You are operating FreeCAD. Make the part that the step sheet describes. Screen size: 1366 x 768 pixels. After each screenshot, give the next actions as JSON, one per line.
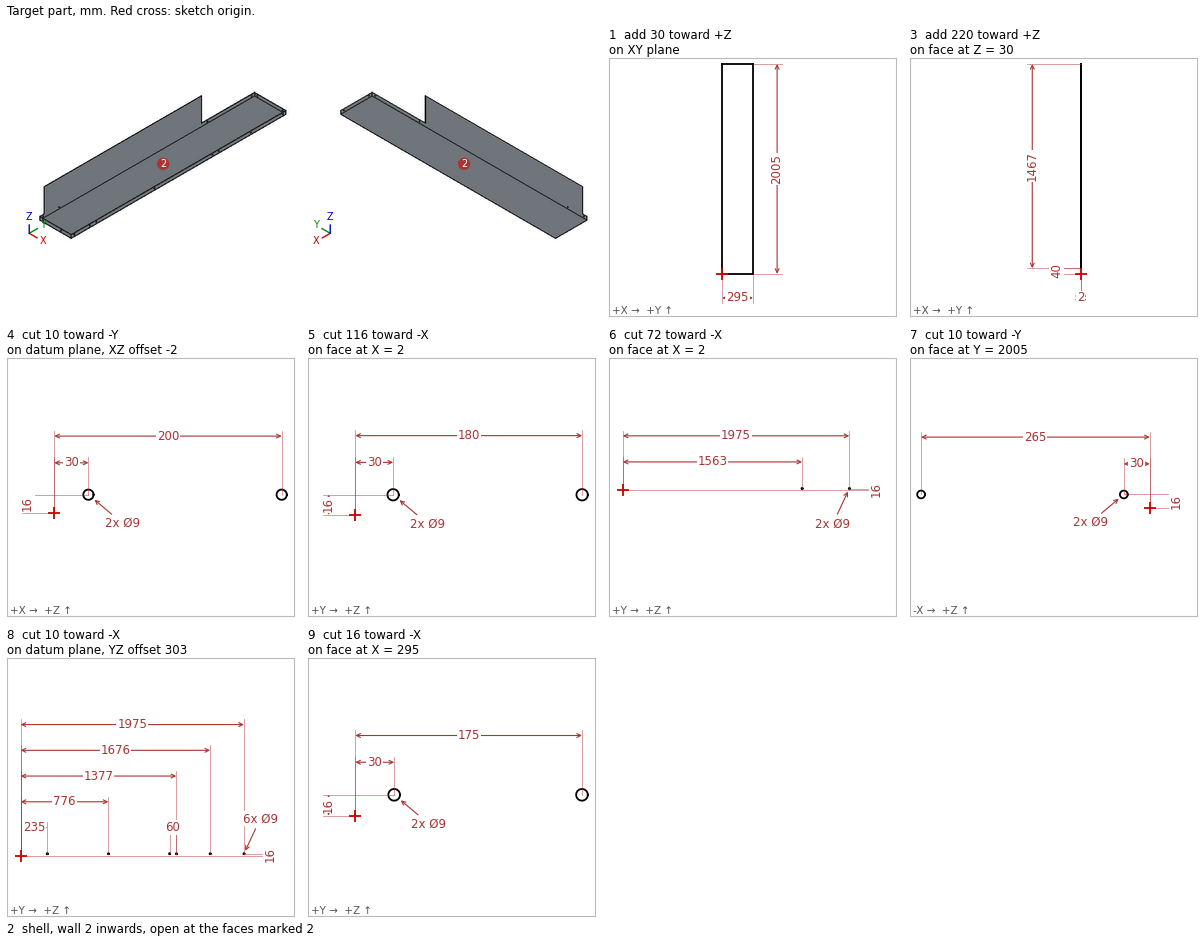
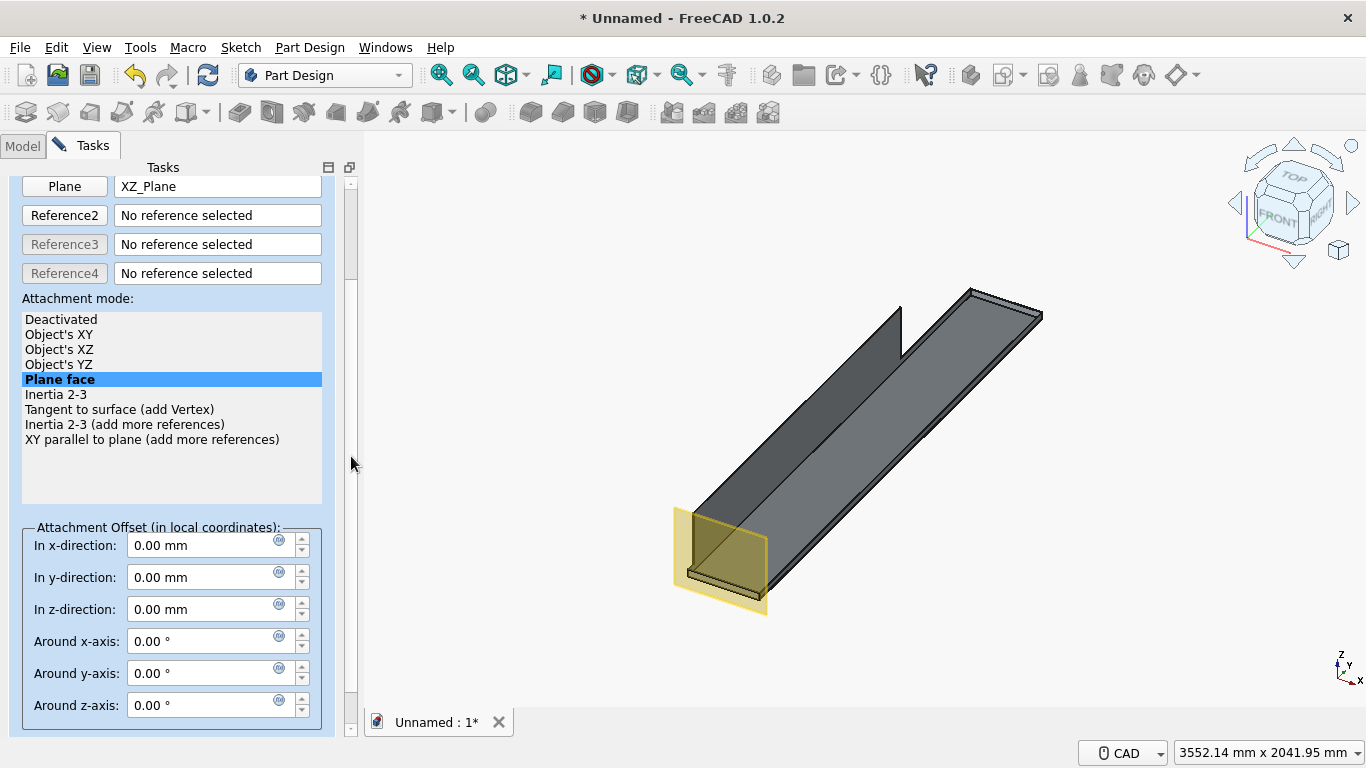
{"action": "triple_click", "coordinate": [210, 609]}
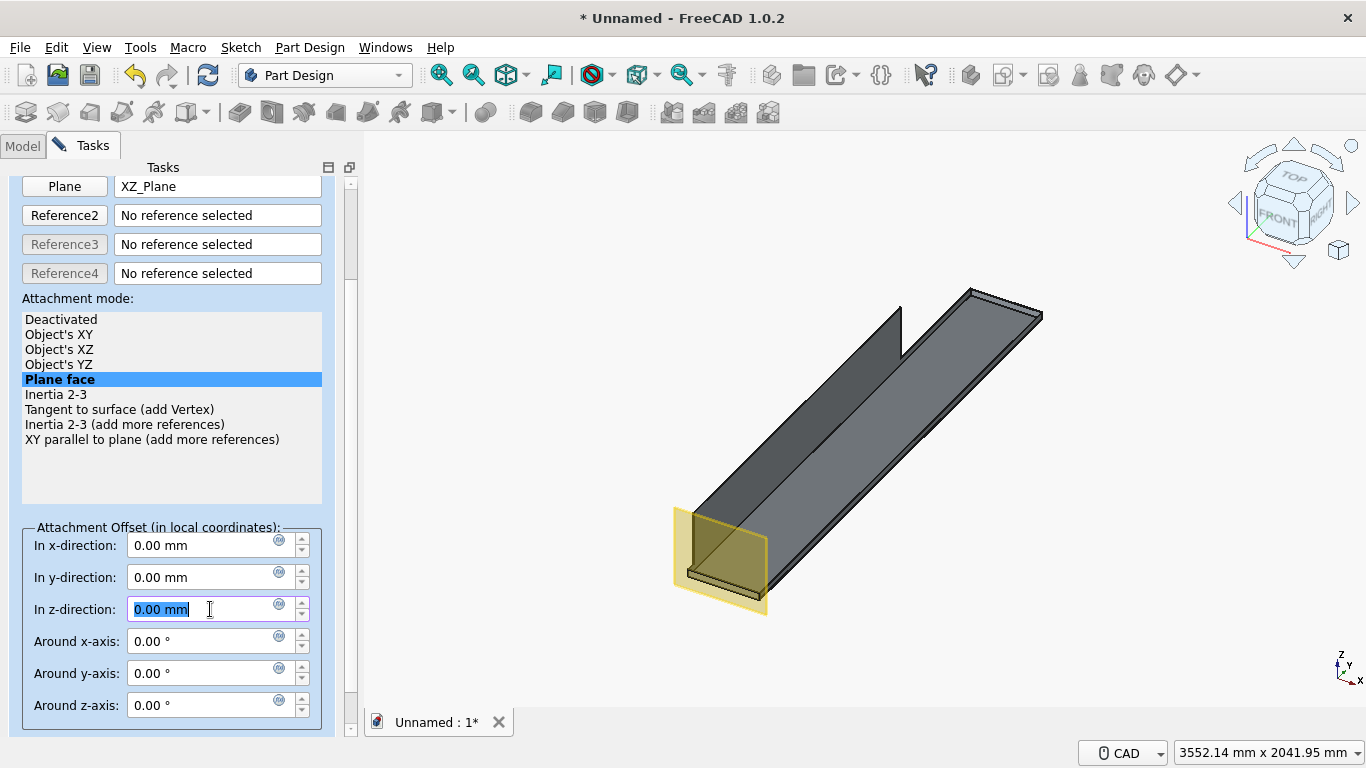
{"action": "type", "text": "-2"}
{"action": "key", "text": "Tab"}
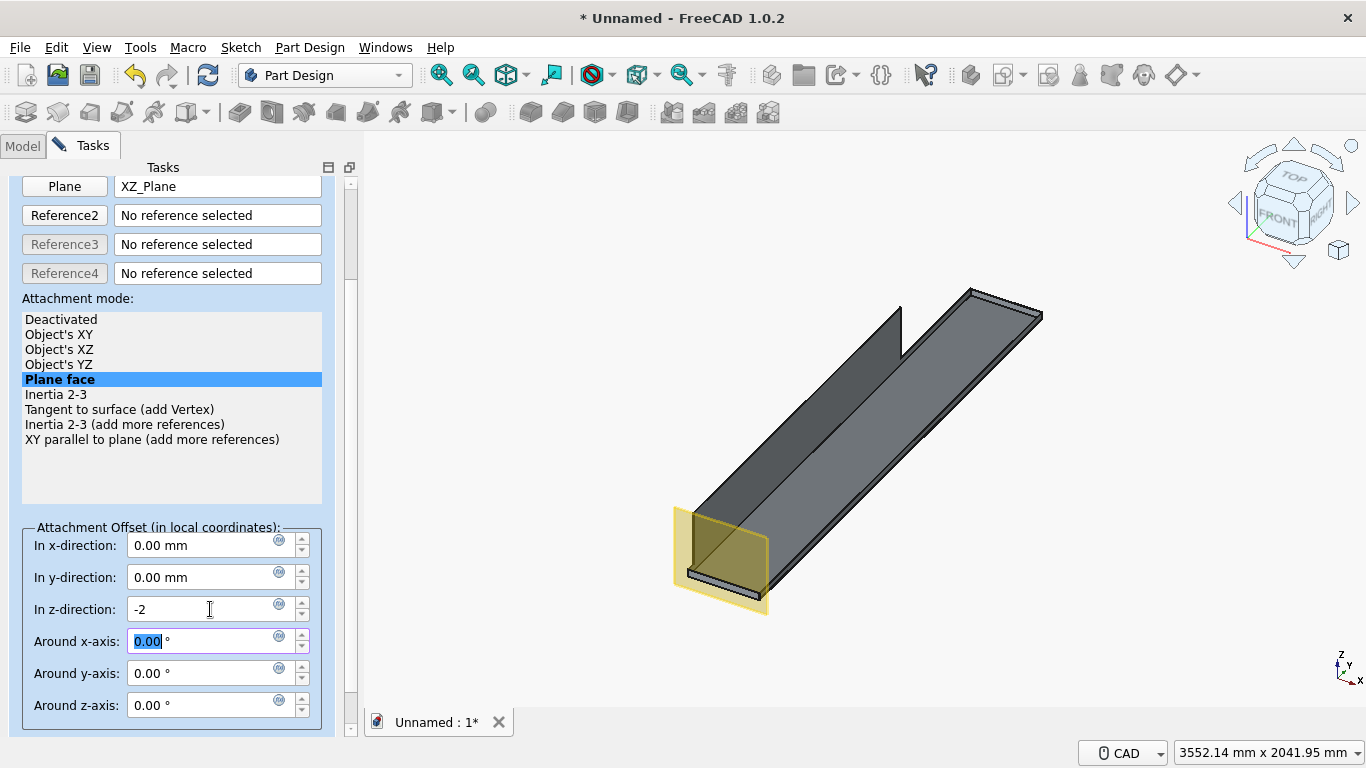
{"action": "scroll", "coordinate": [351, 456], "scroll_direction": "up", "scroll_amount": 3}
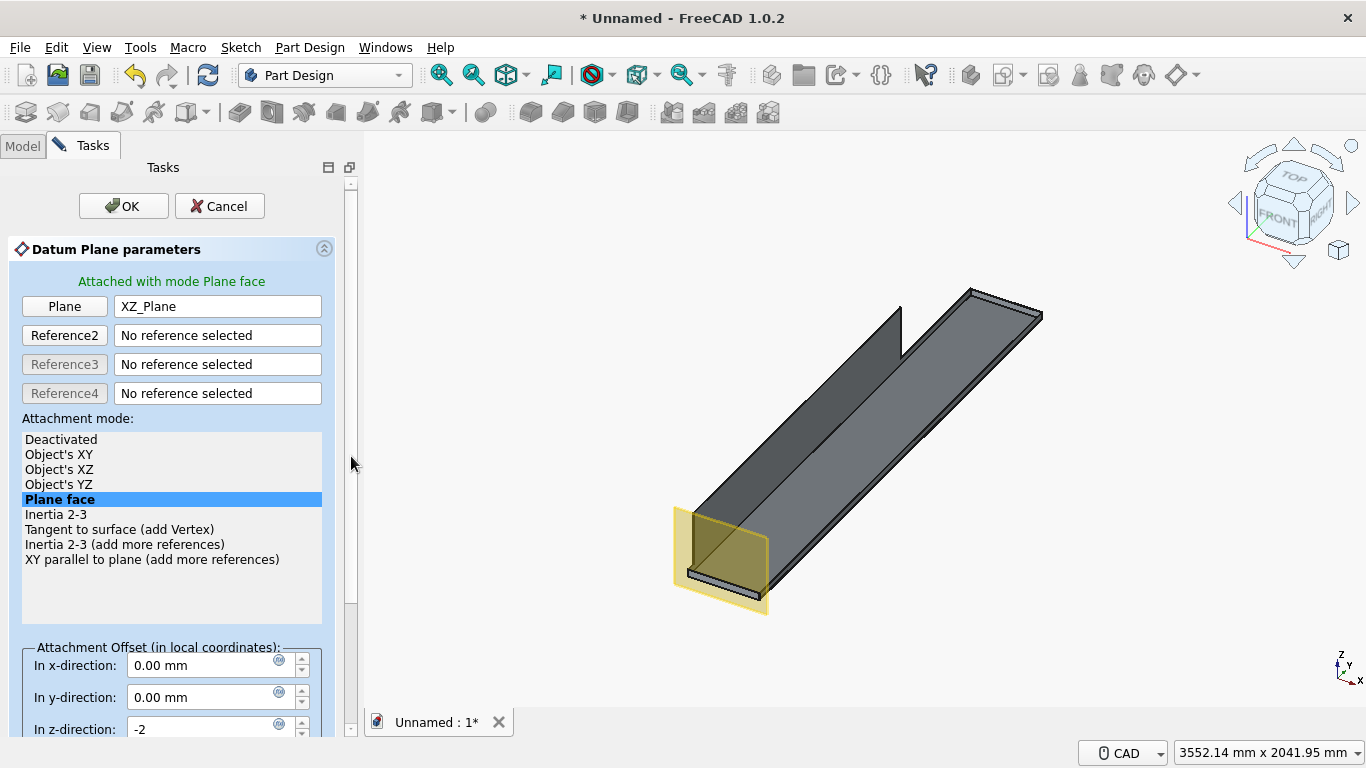
{"action": "left_click", "coordinate": [124, 206]}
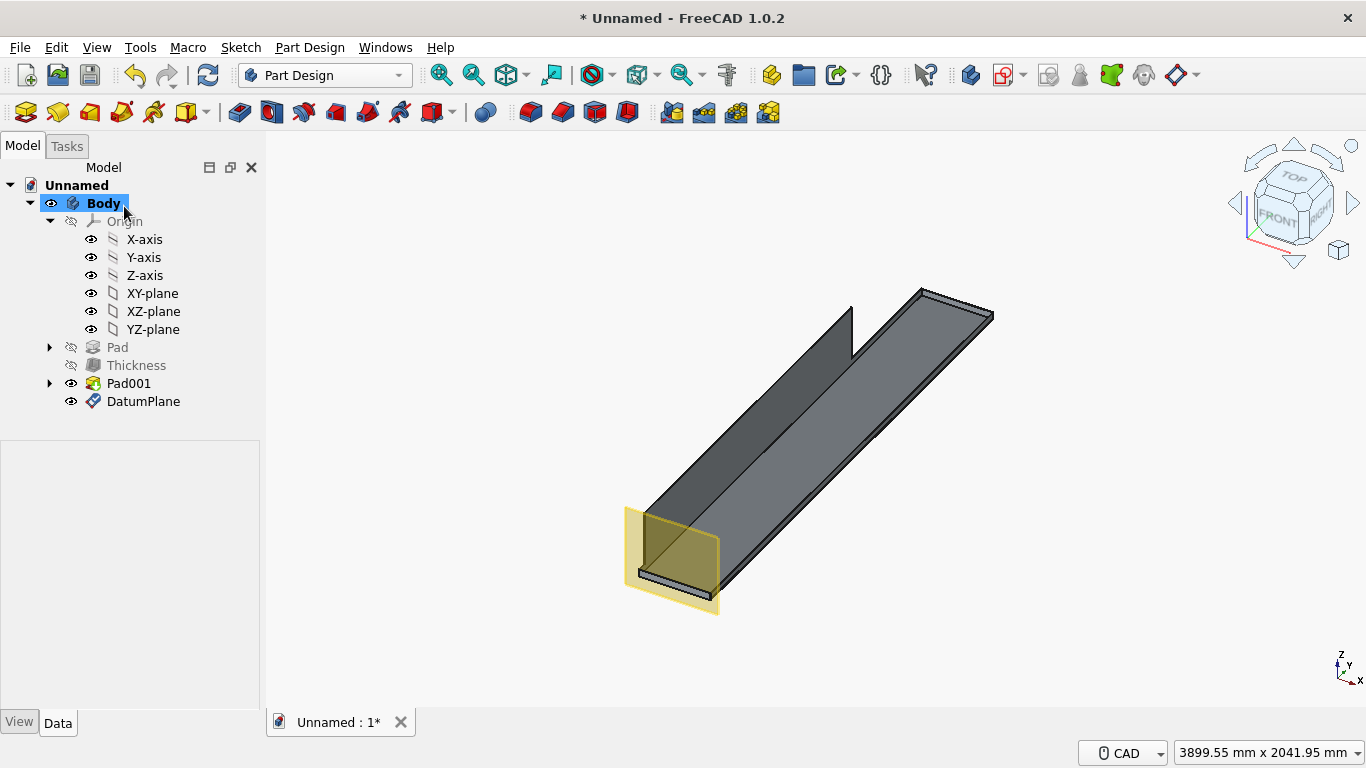
{"action": "left_click", "coordinate": [116, 401]}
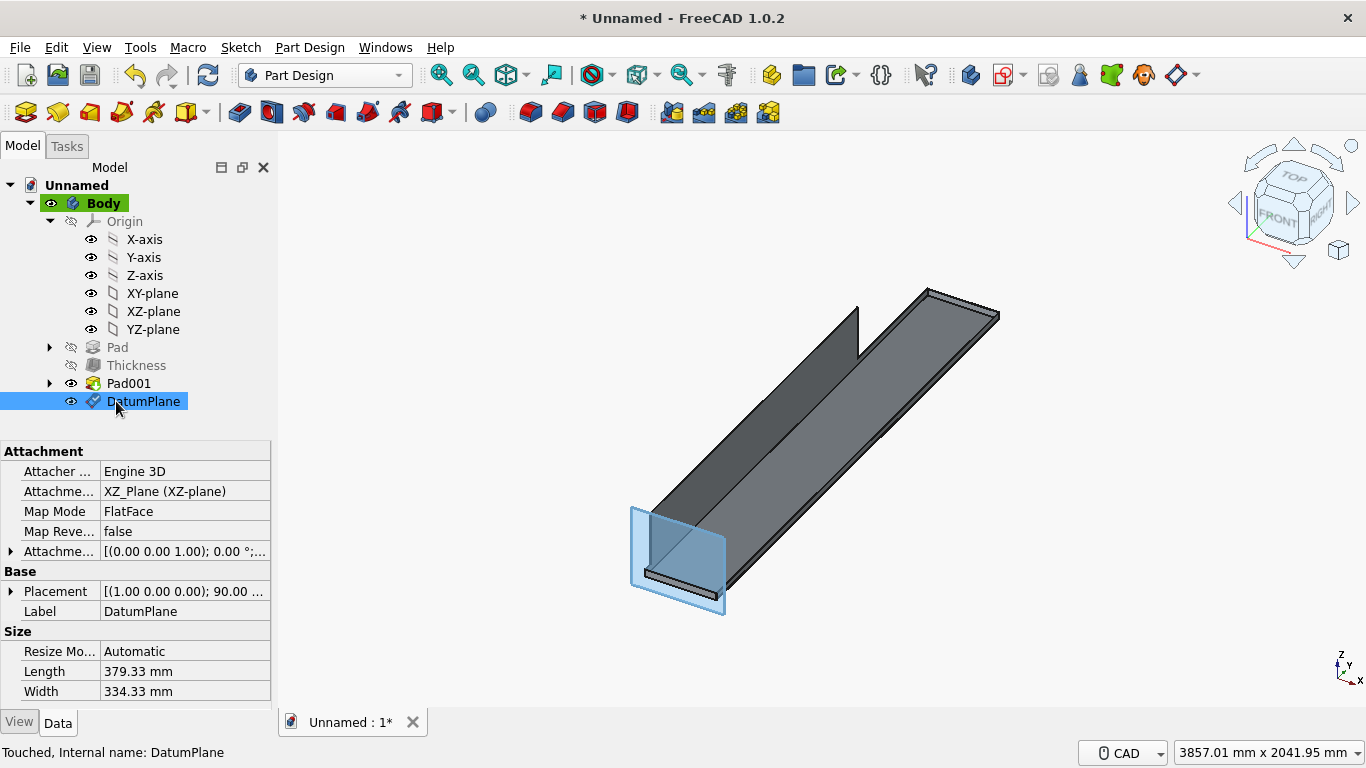
{"action": "left_click", "coordinate": [1004, 76]}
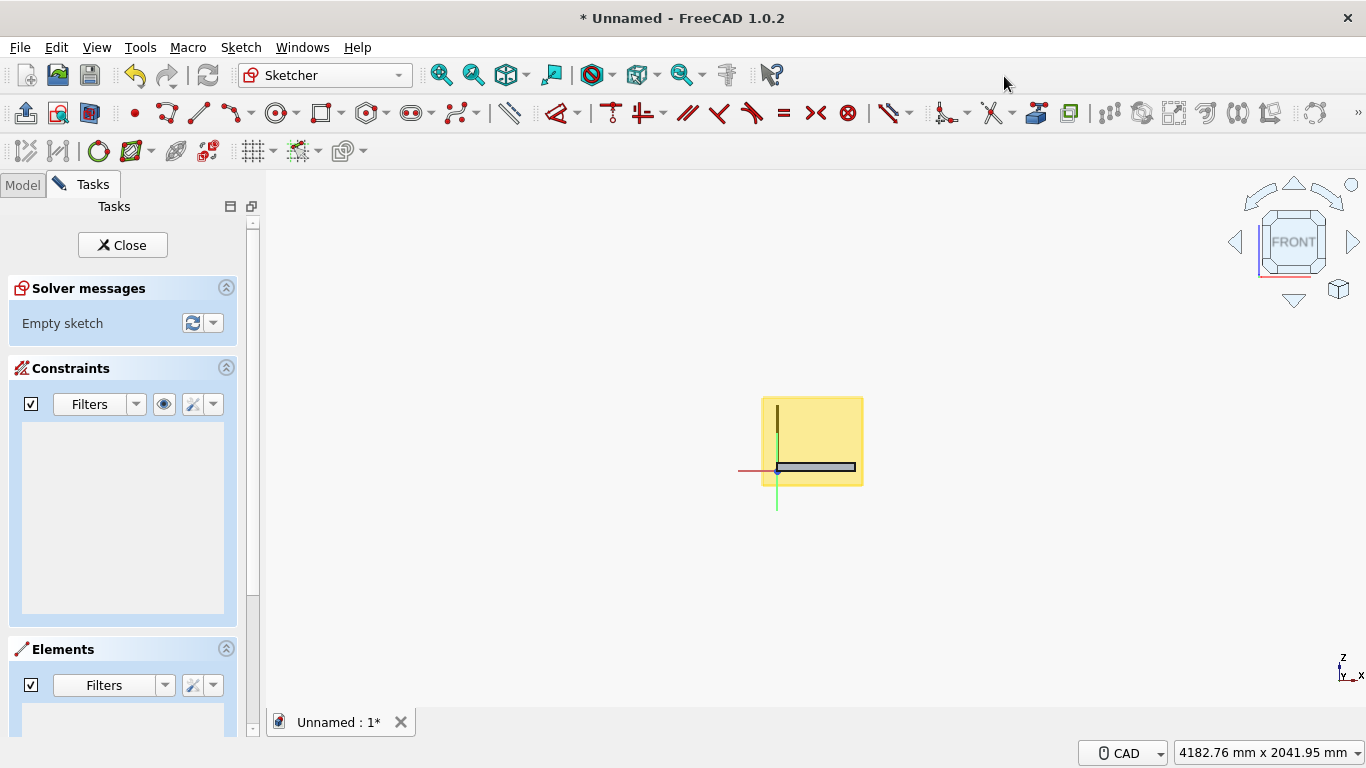
{"action": "left_click", "coordinate": [90, 114]}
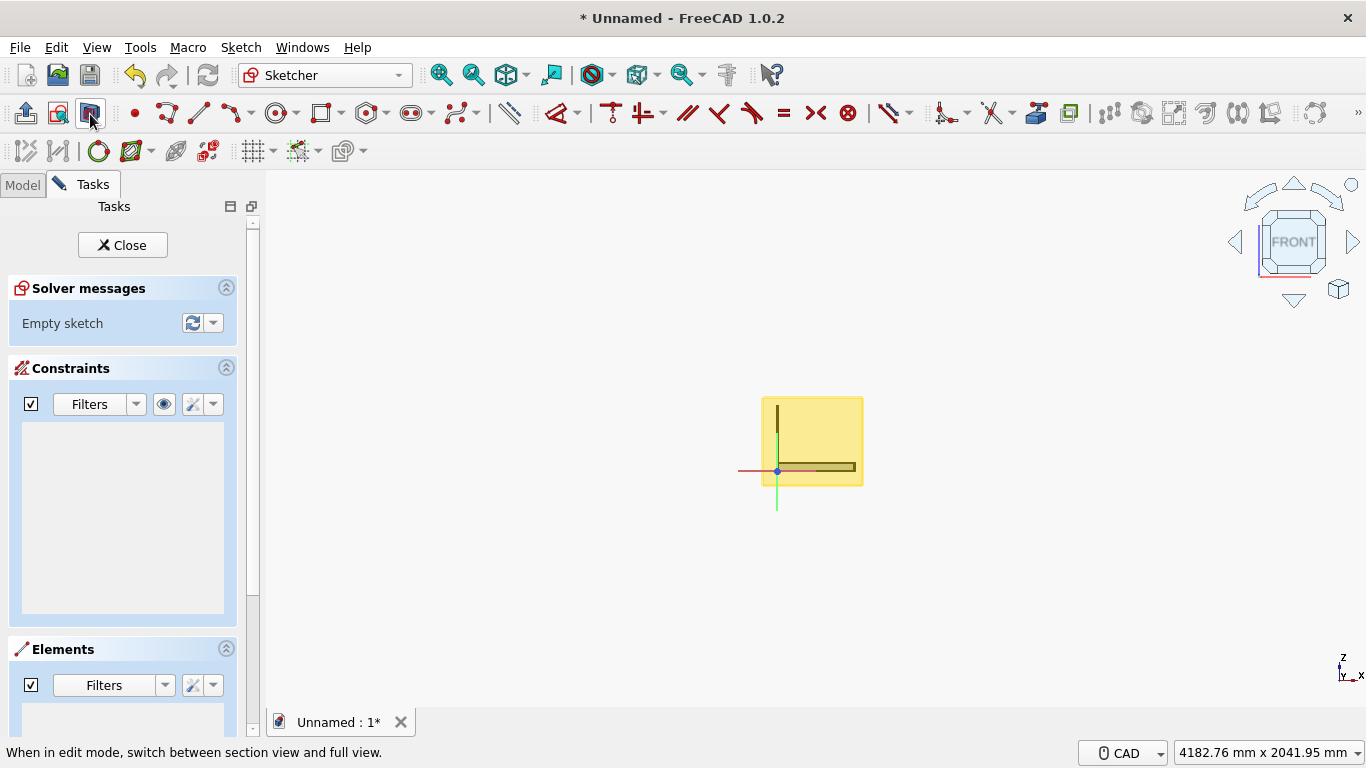
{"action": "scroll", "coordinate": [810, 472], "scroll_direction": "up", "scroll_amount": 12}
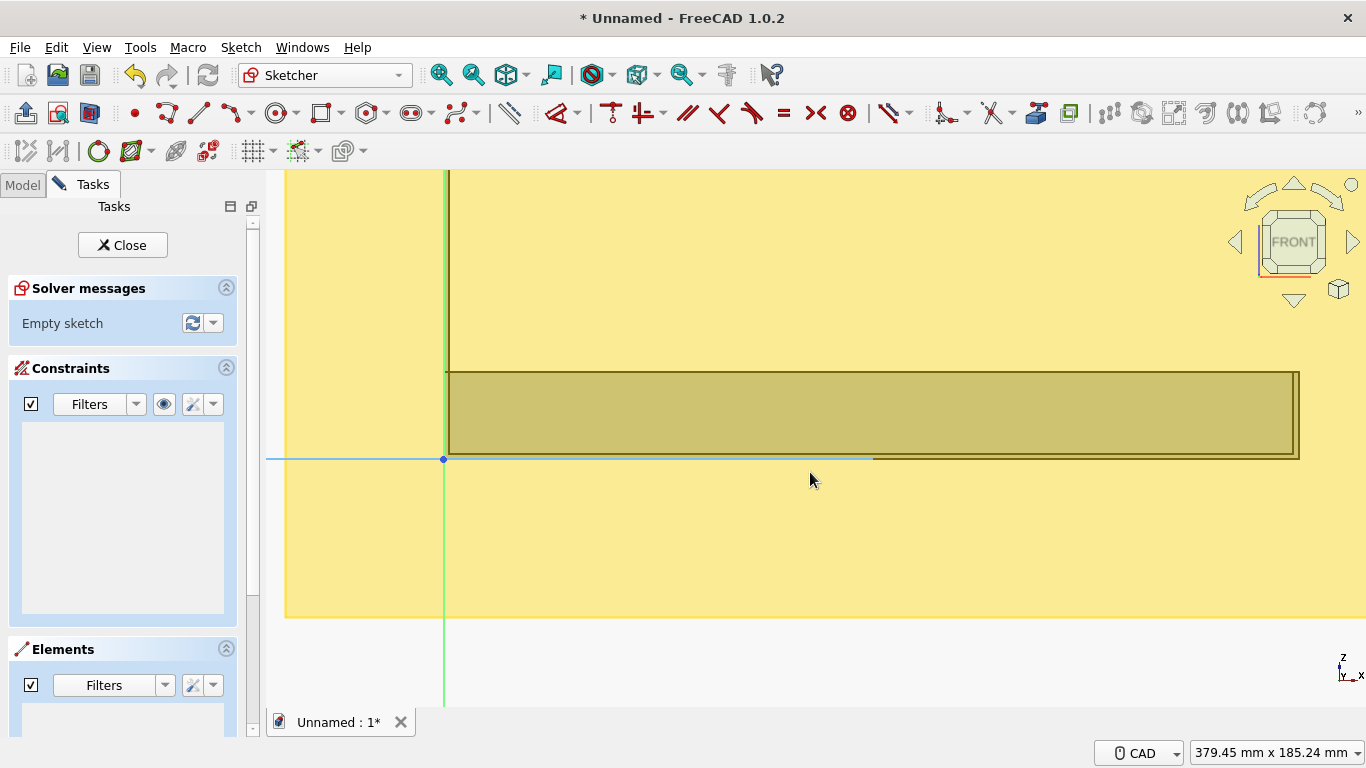
{"action": "left_click", "coordinate": [276, 114]}